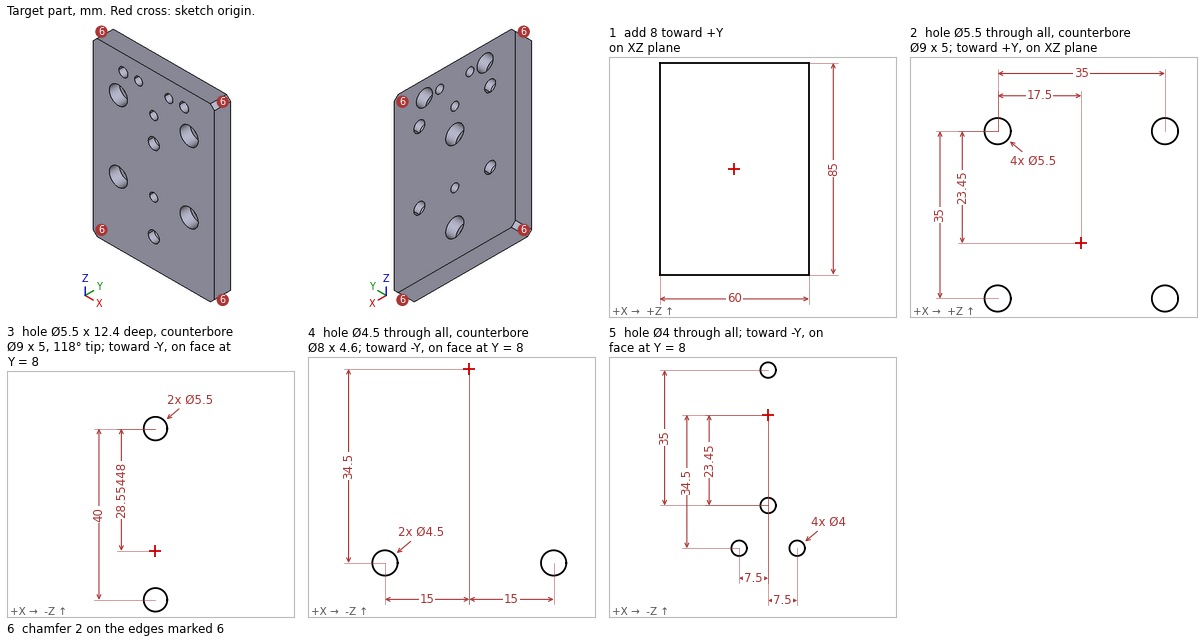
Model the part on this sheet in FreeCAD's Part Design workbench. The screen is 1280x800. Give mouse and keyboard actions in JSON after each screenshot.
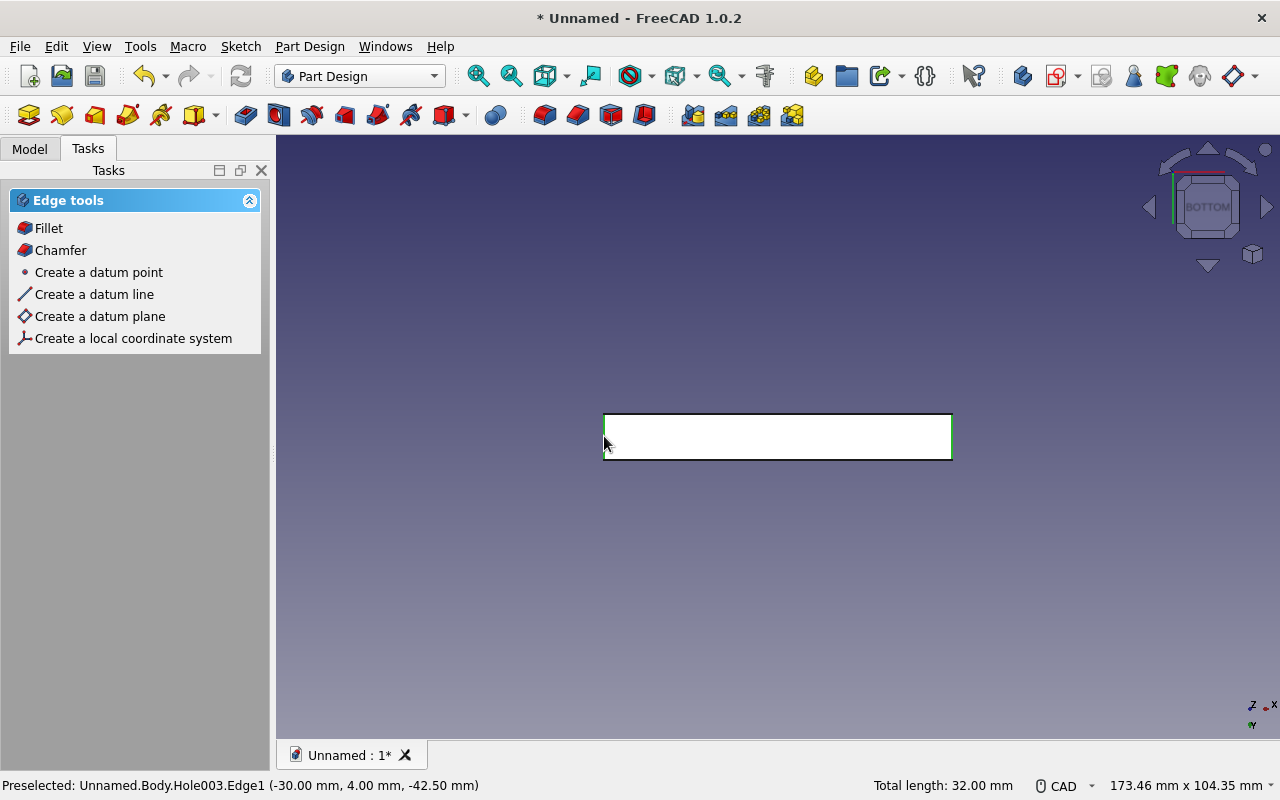
{"action": "left_click", "coordinate": [578, 116]}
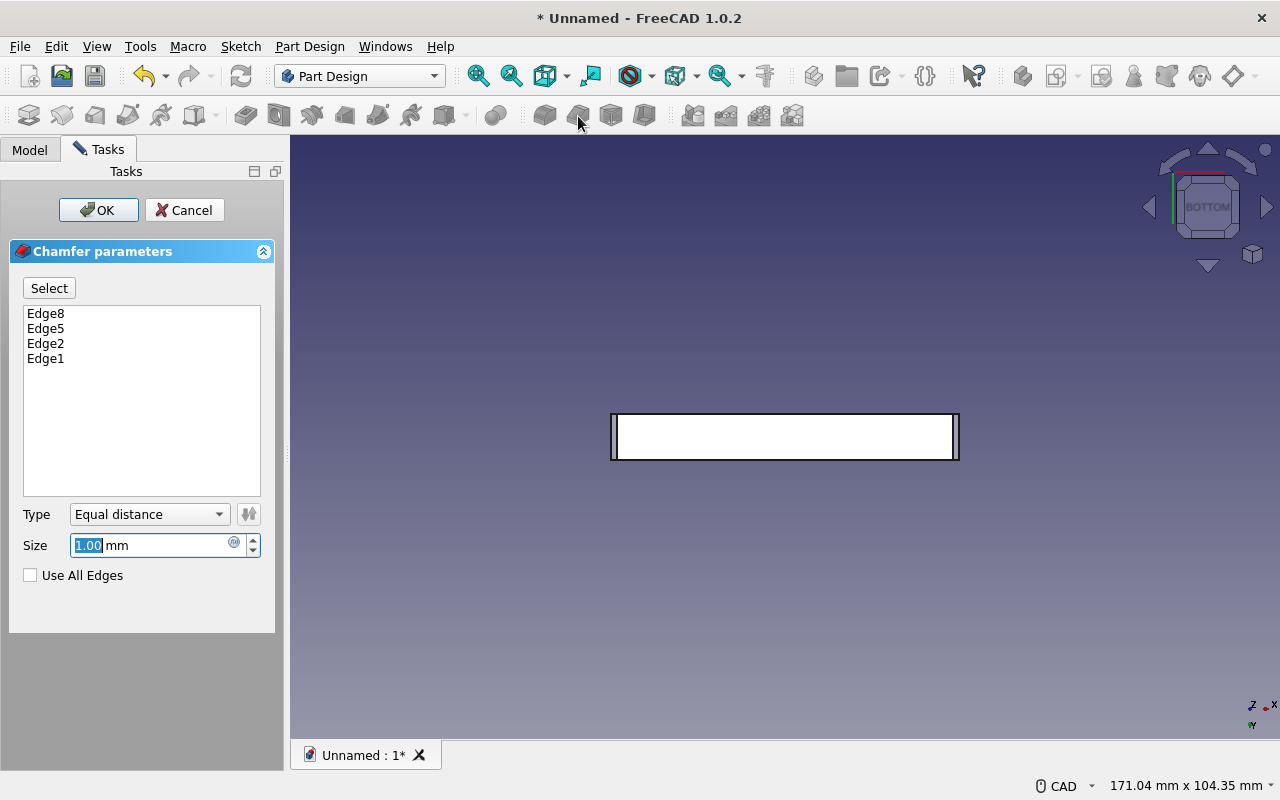
{"action": "type", "text": "2"}
{"action": "key", "text": "Tab"}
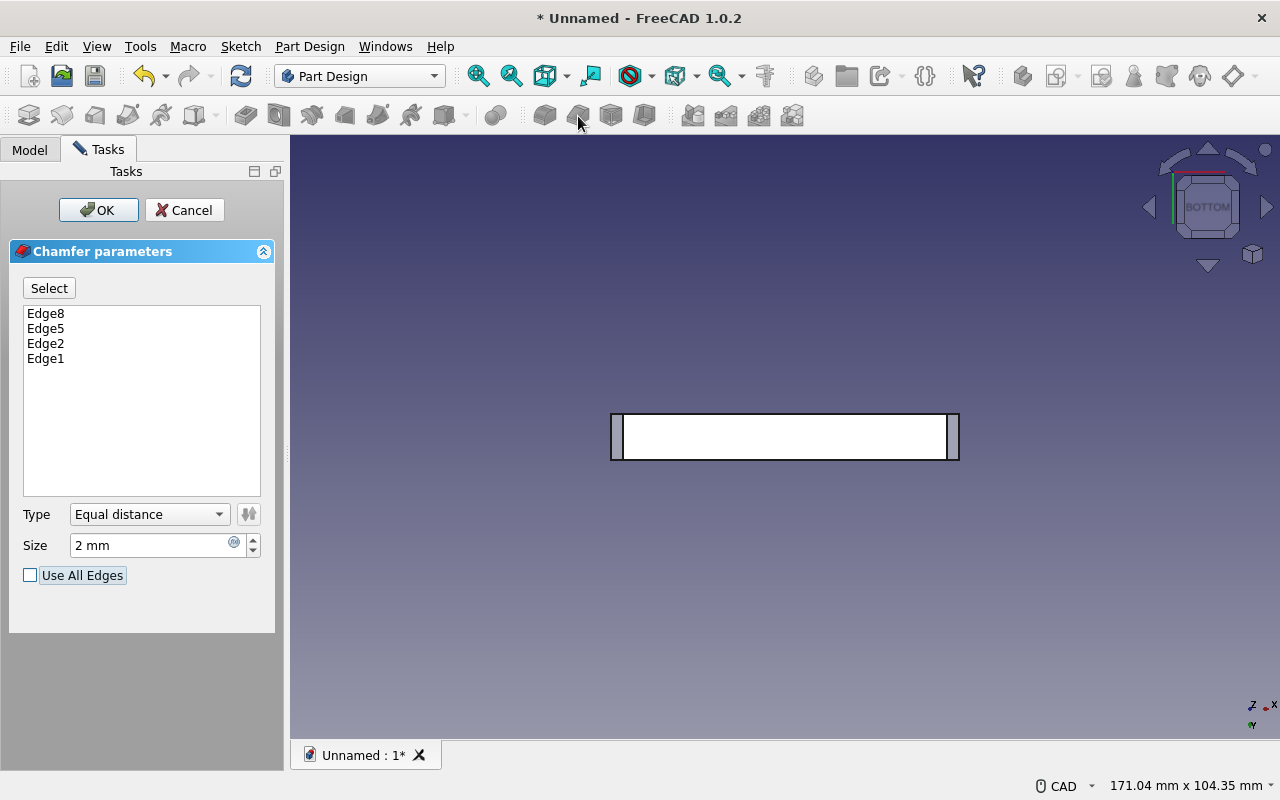
{"action": "left_click", "coordinate": [99, 210]}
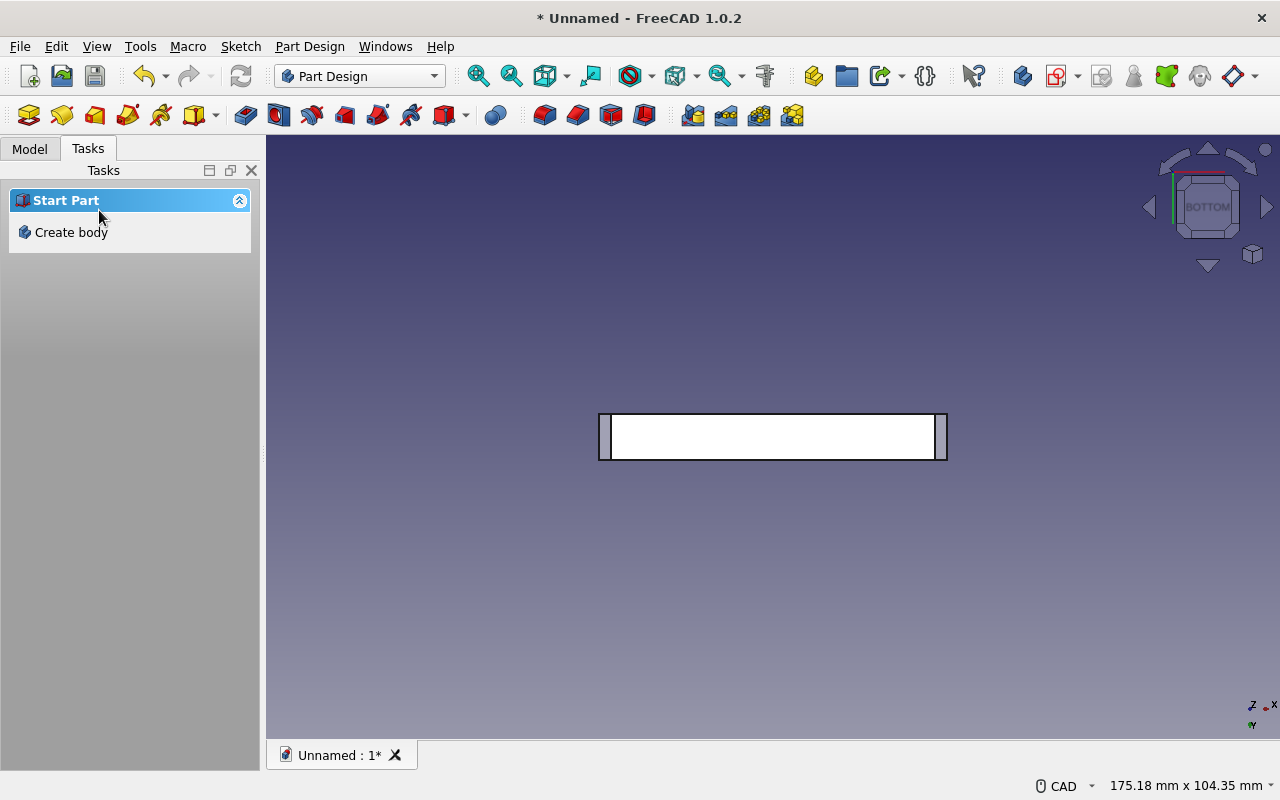
{"action": "key", "text": "0"}